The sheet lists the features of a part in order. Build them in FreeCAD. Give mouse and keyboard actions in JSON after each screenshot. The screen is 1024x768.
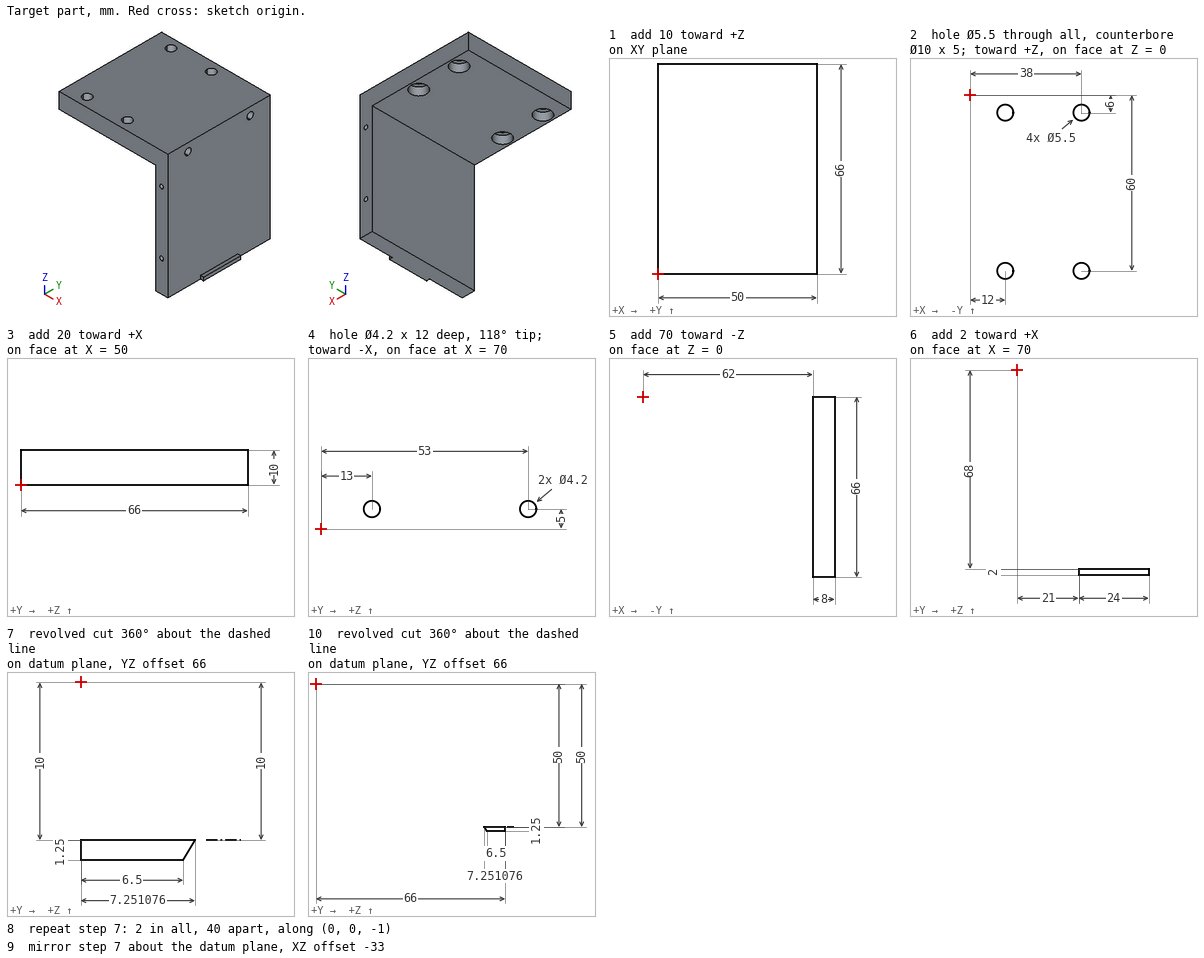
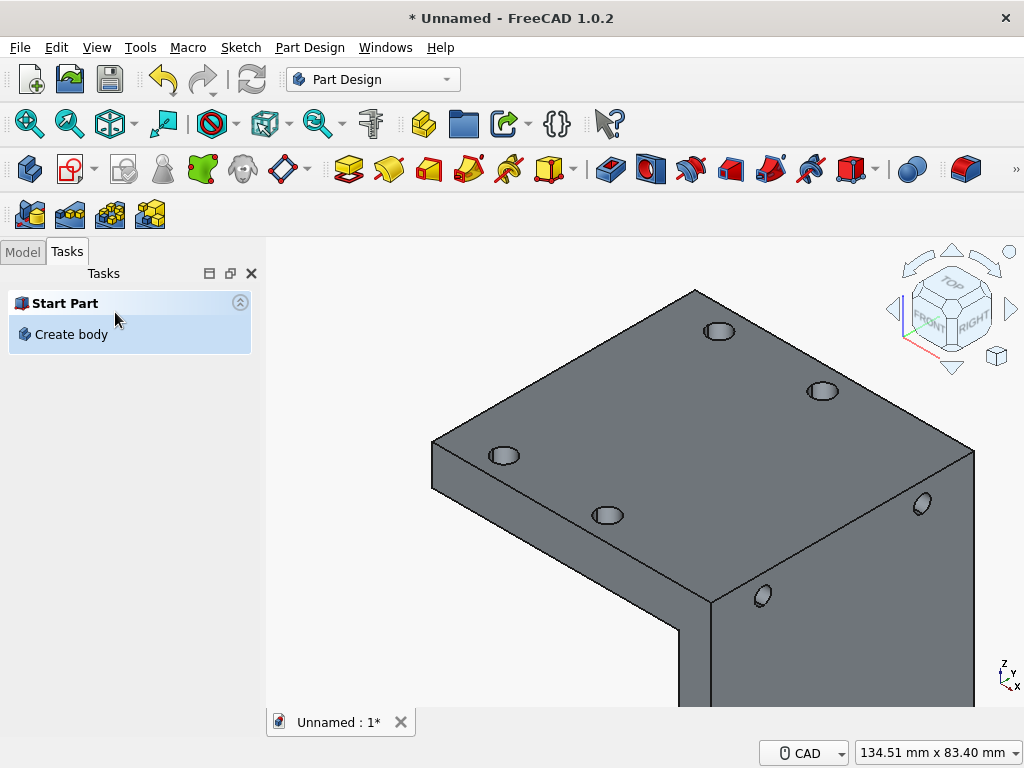
{"action": "left_click", "coordinate": [30, 124]}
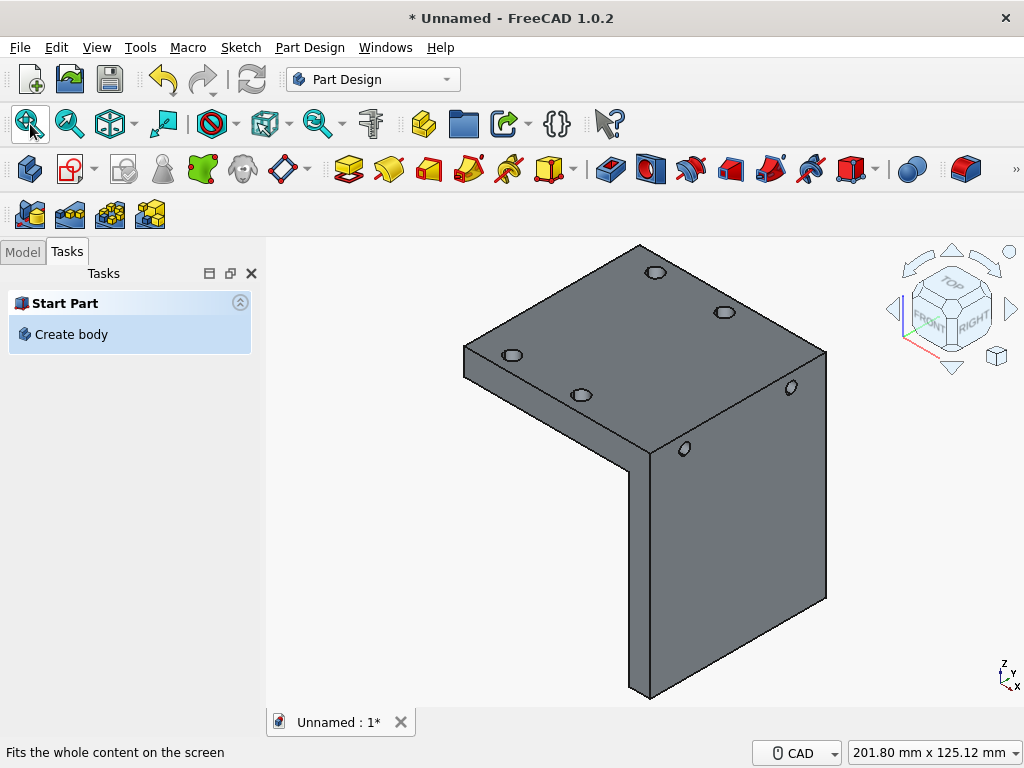
{"action": "left_click", "coordinate": [738, 525]}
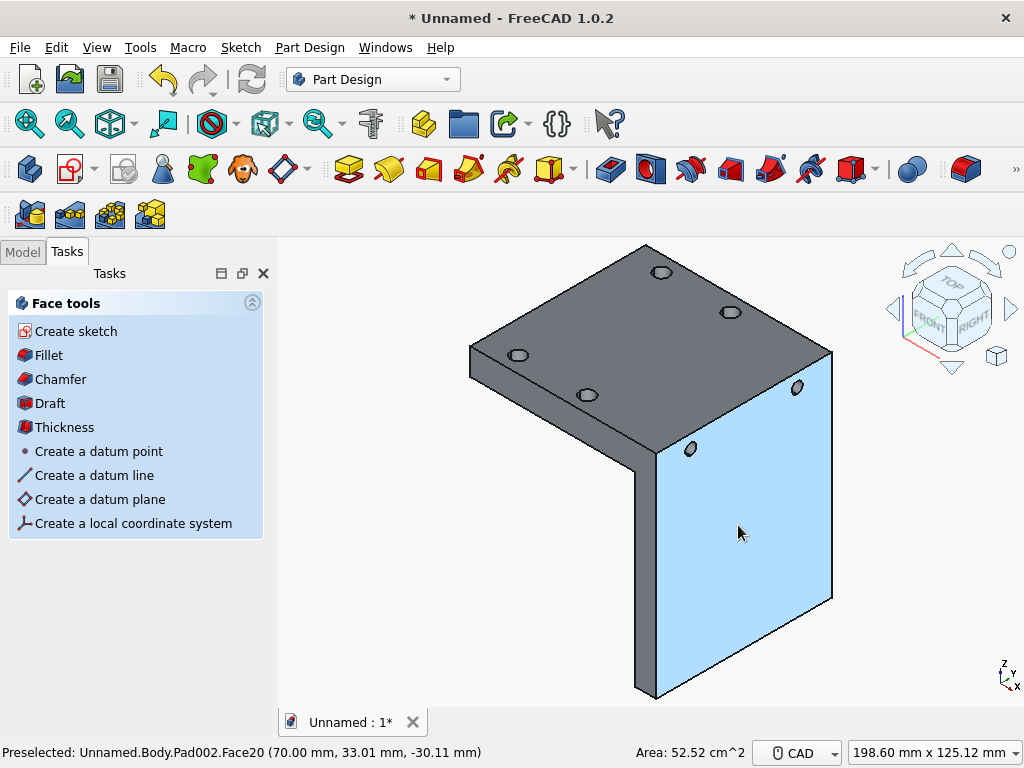
{"action": "left_click", "coordinate": [70, 170]}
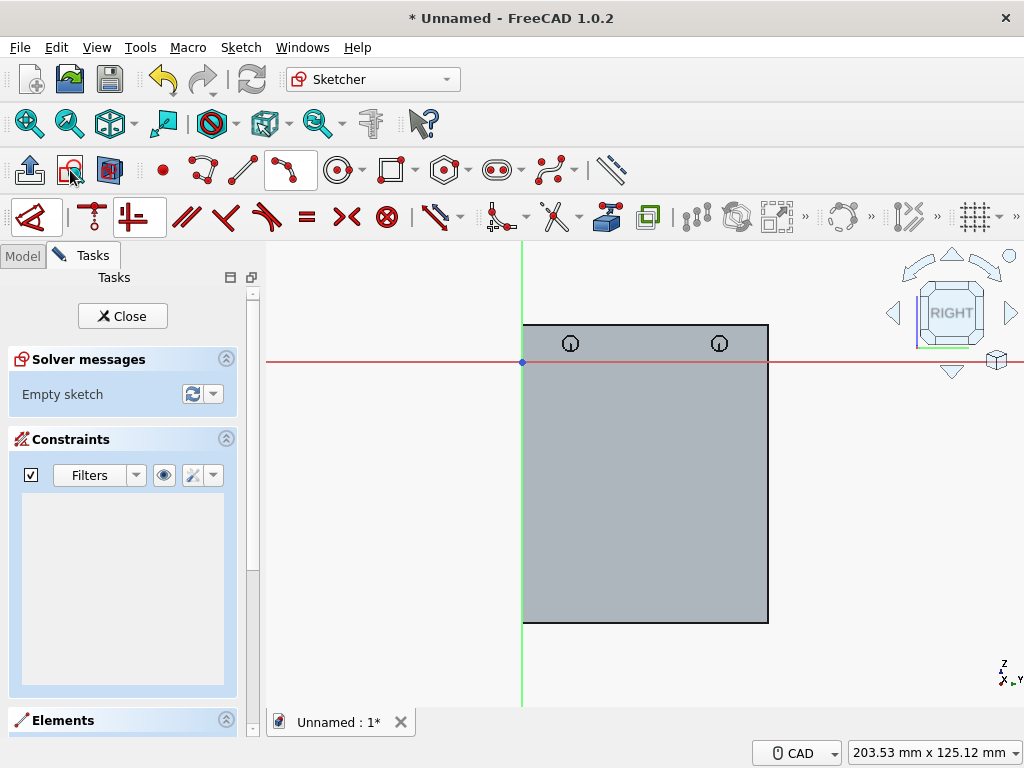
{"action": "scroll", "coordinate": [667, 667], "scroll_direction": "up", "scroll_amount": 7}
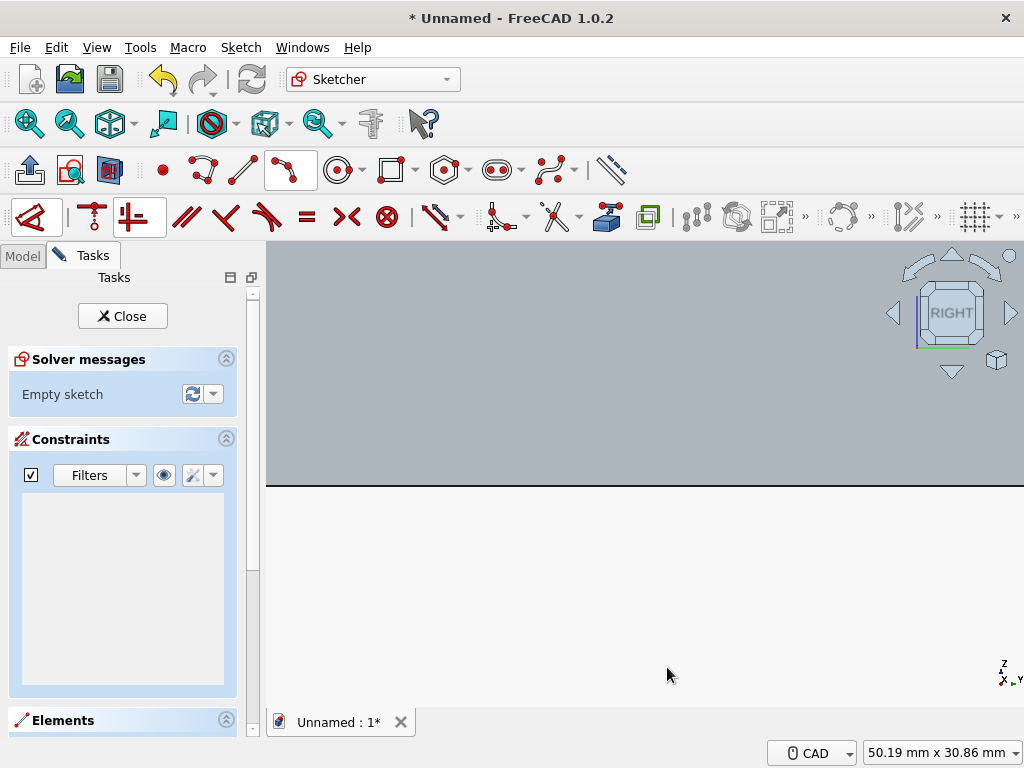
{"action": "left_click", "coordinate": [392, 170]}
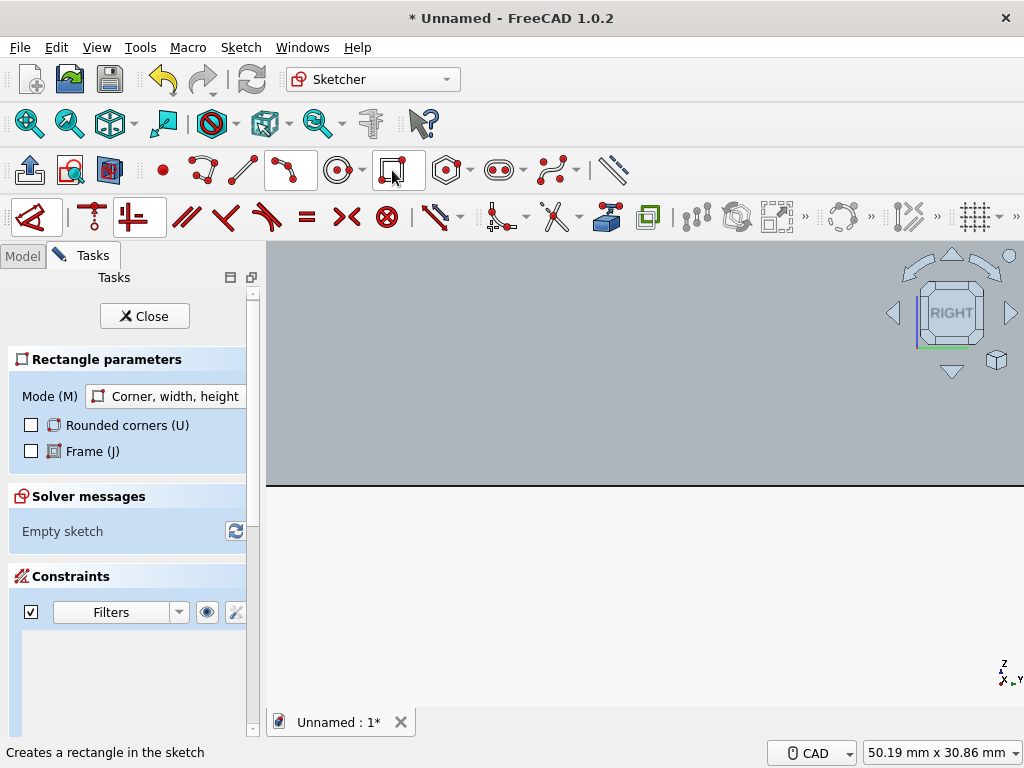
{"action": "left_click", "coordinate": [395, 455]}
{"action": "left_click", "coordinate": [757, 486]}
{"action": "key", "text": "Escape"}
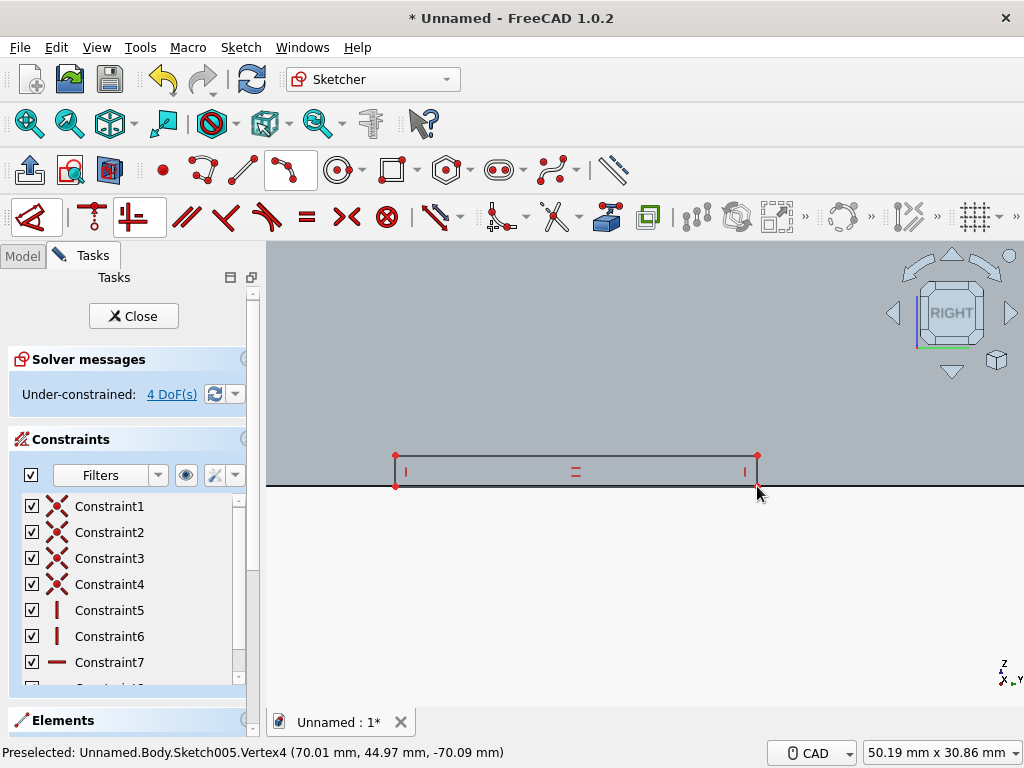
{"action": "scroll", "coordinate": [395, 465], "scroll_direction": "up", "scroll_amount": 2}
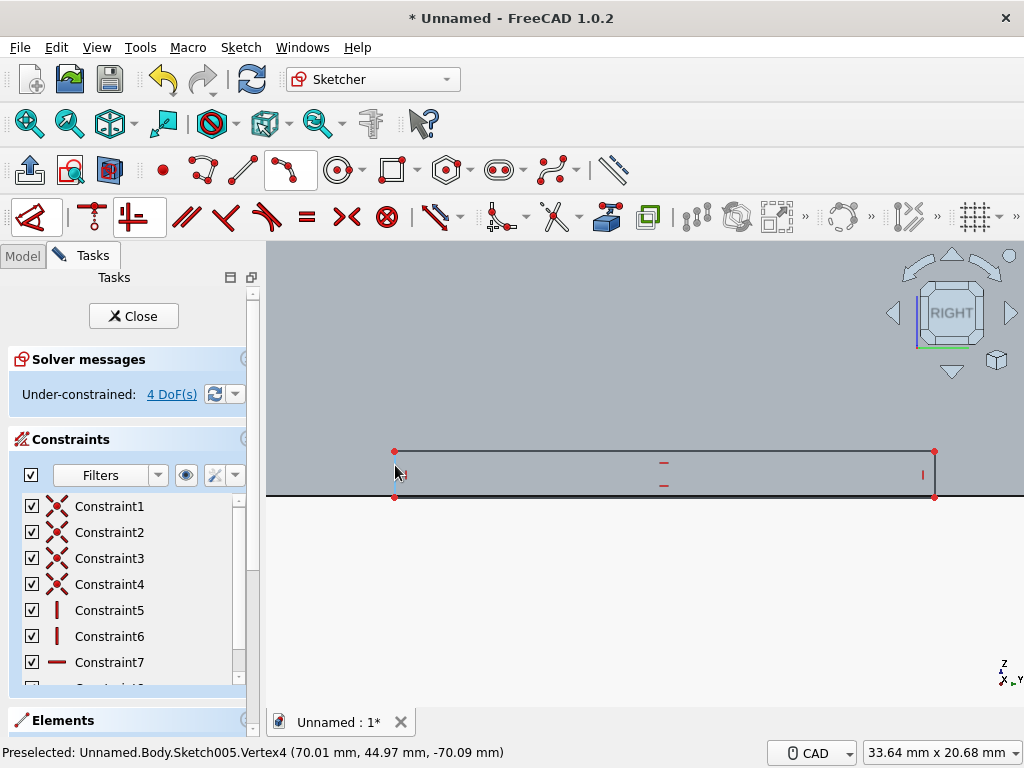
{"action": "left_click", "coordinate": [395, 465]}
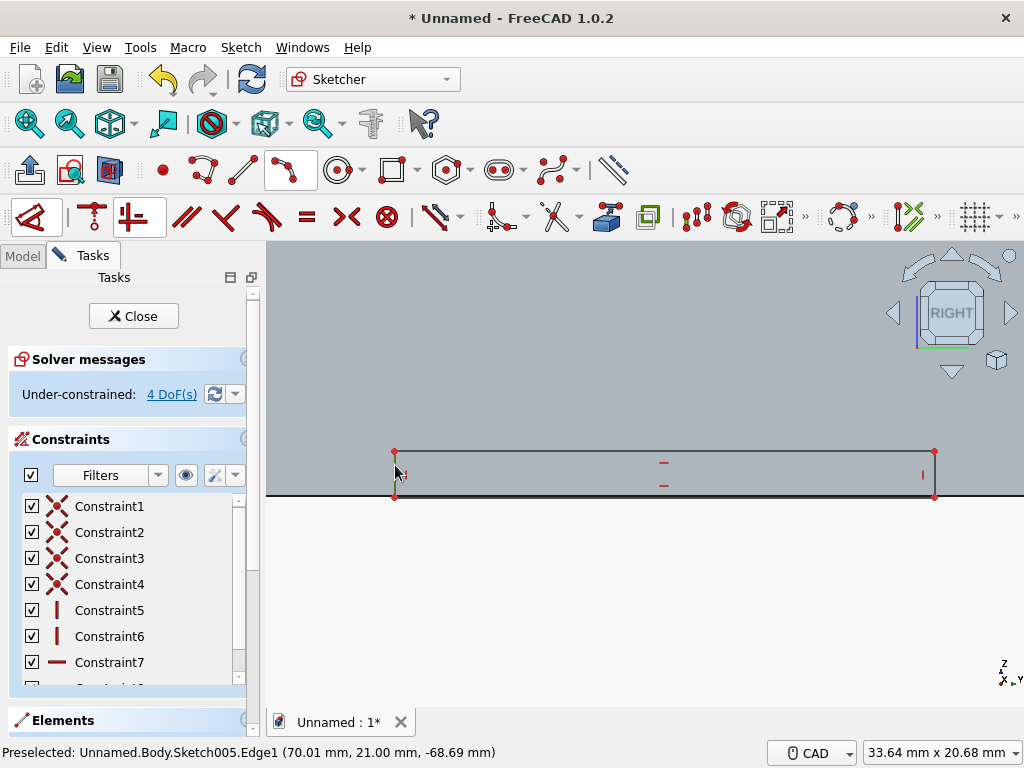
{"action": "key", "text": "i"}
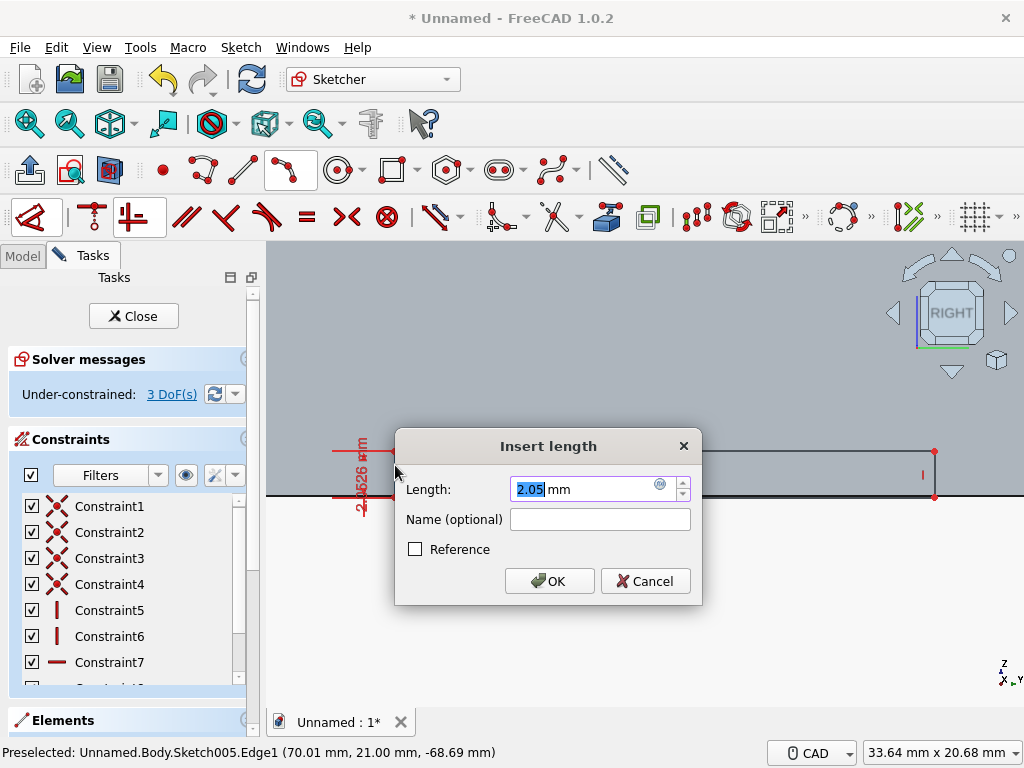
{"action": "type", "text": "2"}
{"action": "key", "text": "Return"}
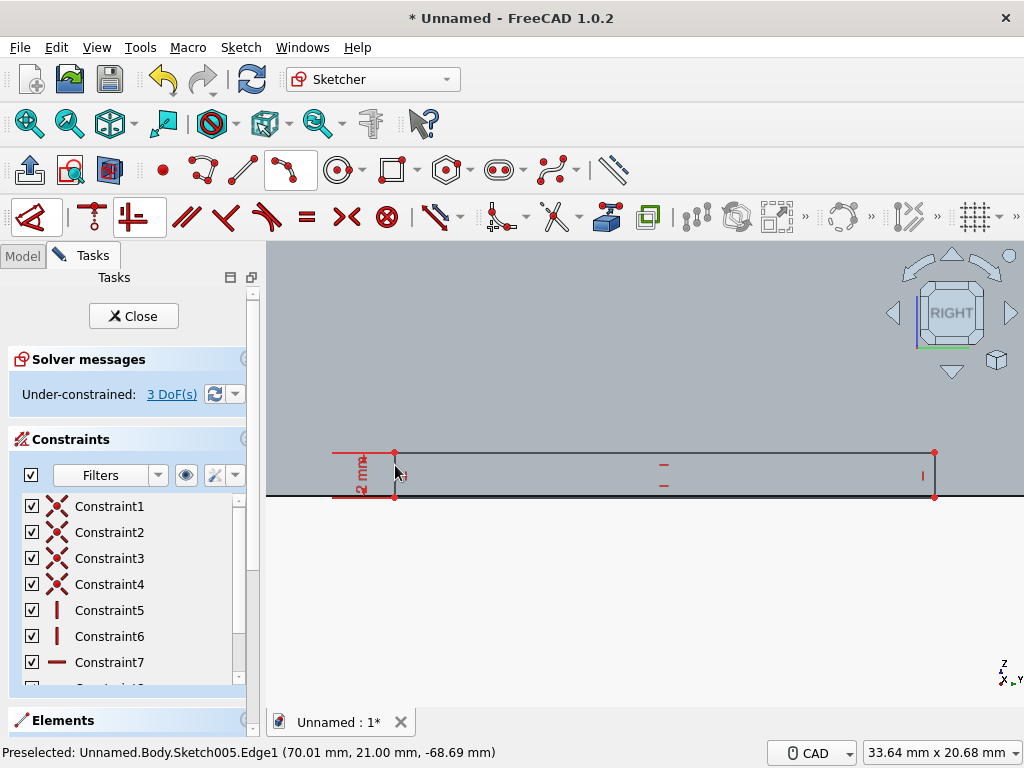
{"action": "left_click", "coordinate": [557, 498]}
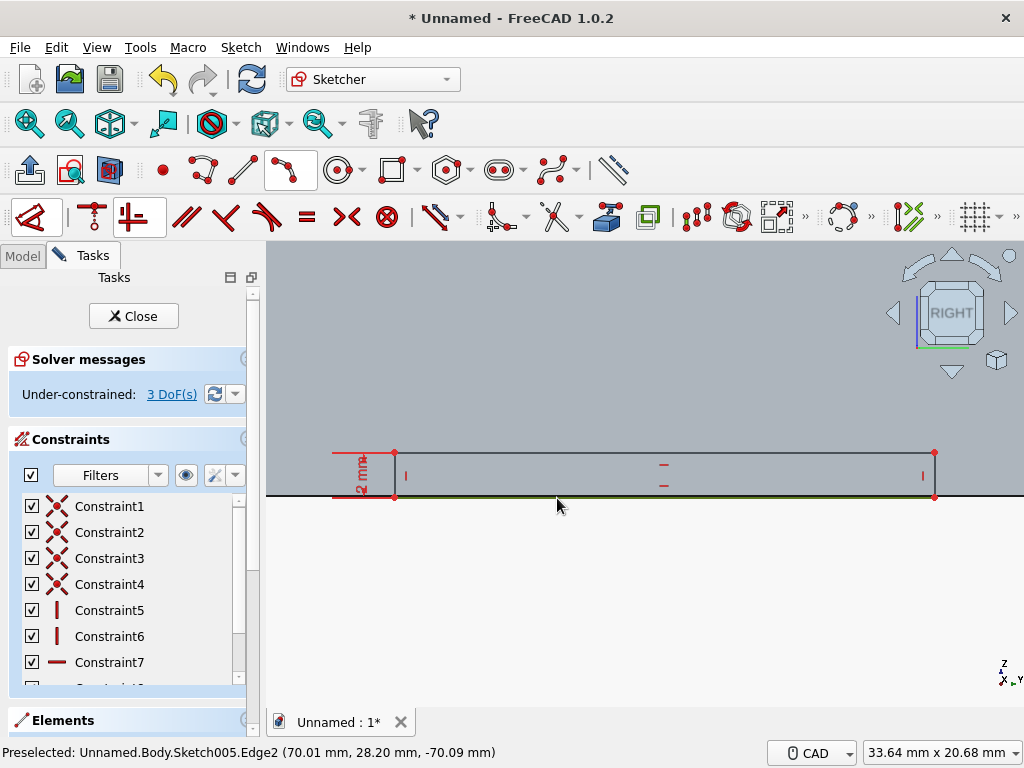
{"action": "left_click", "coordinate": [56, 218]}